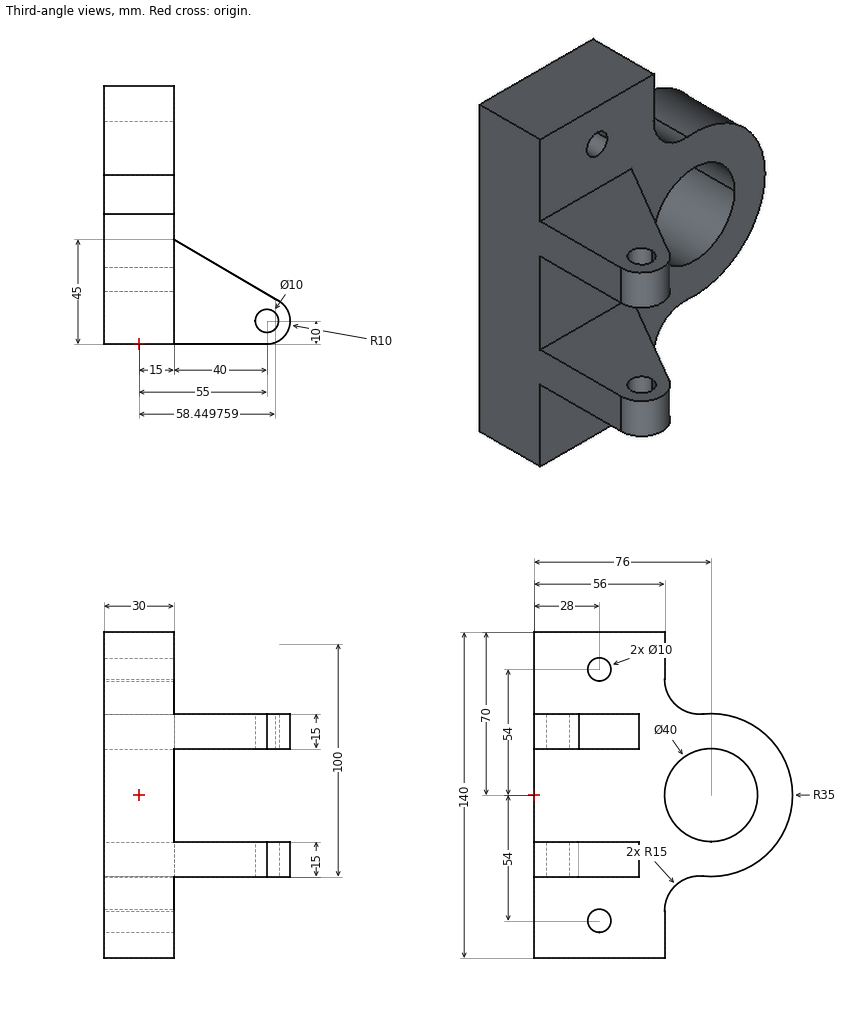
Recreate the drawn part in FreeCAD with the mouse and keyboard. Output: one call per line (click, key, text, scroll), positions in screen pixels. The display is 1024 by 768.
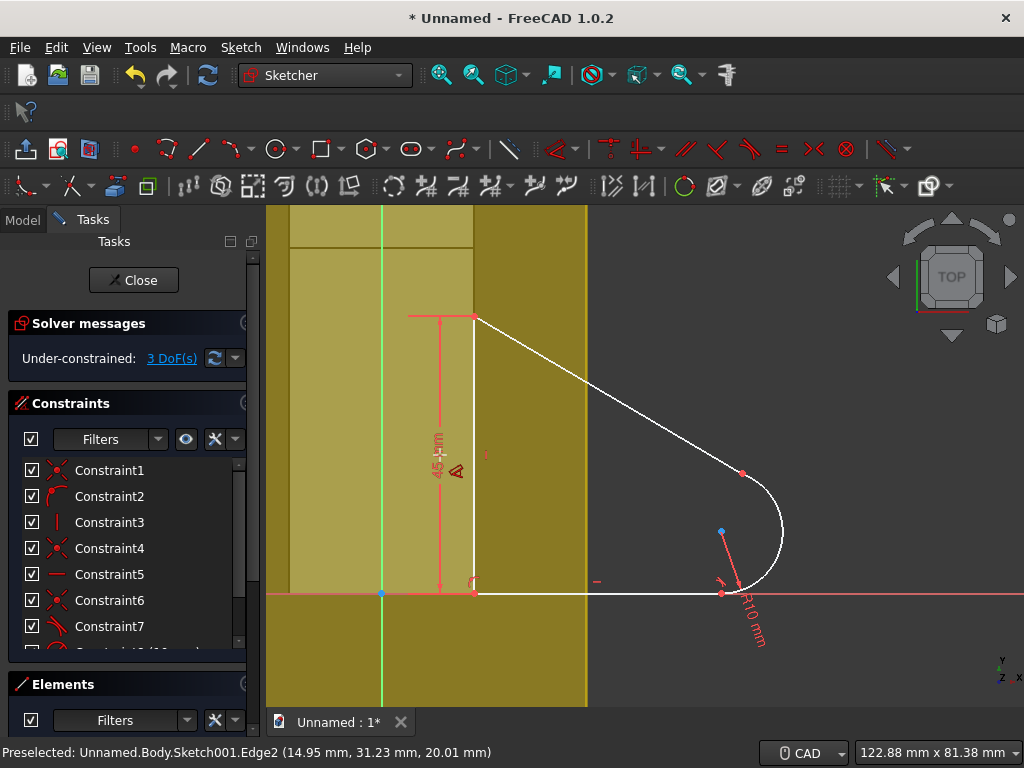
click(548, 594)
click(598, 628)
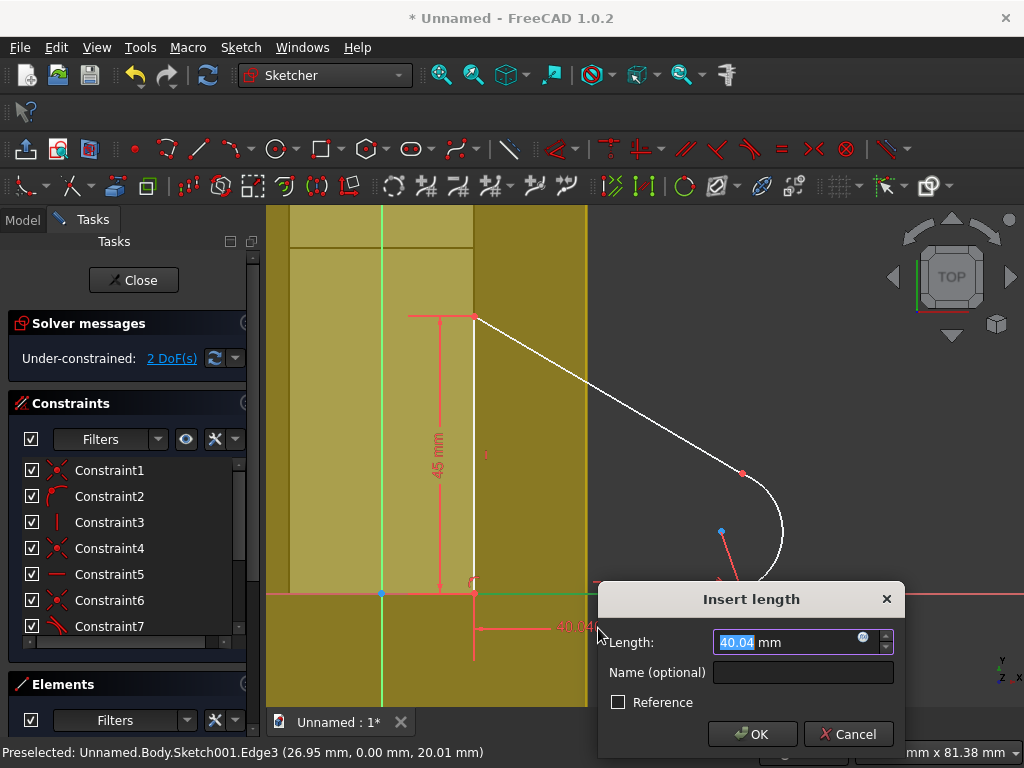
text(40)
key(Return)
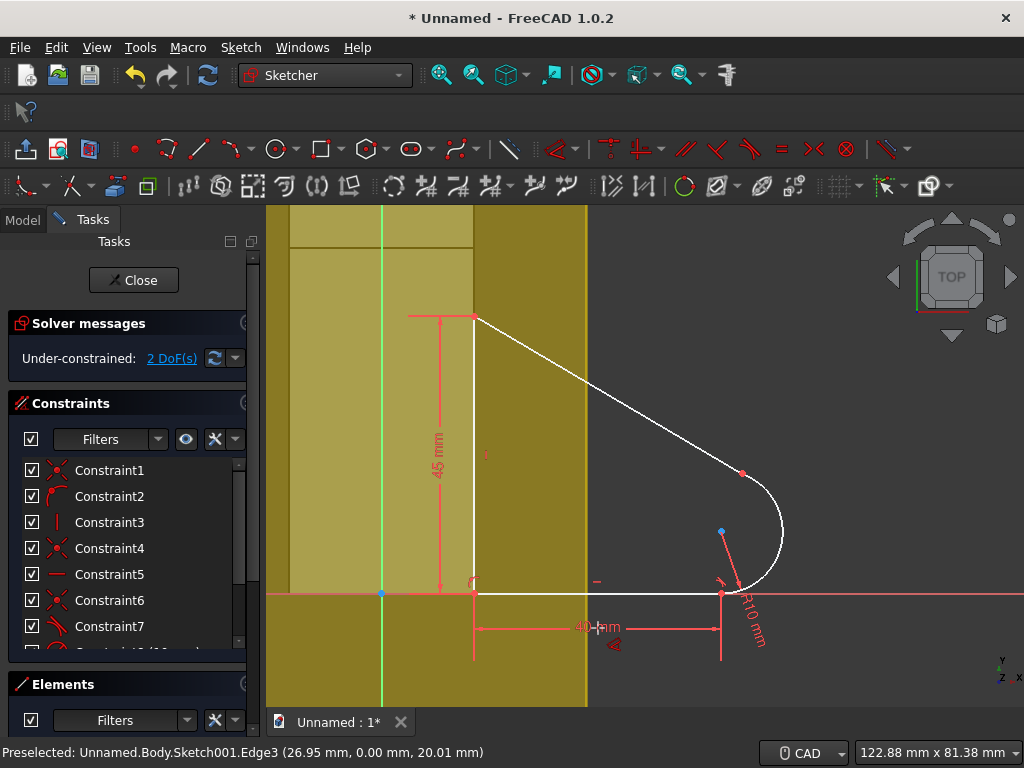
click(474, 316)
click(428, 628)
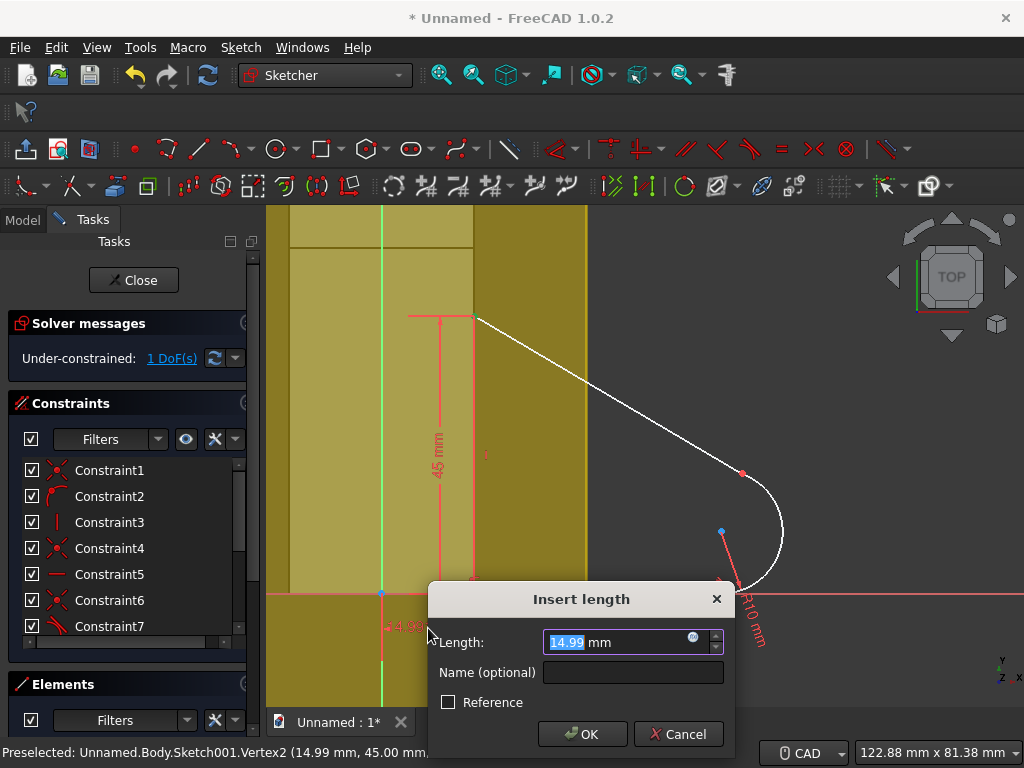
text(15)
key(Return)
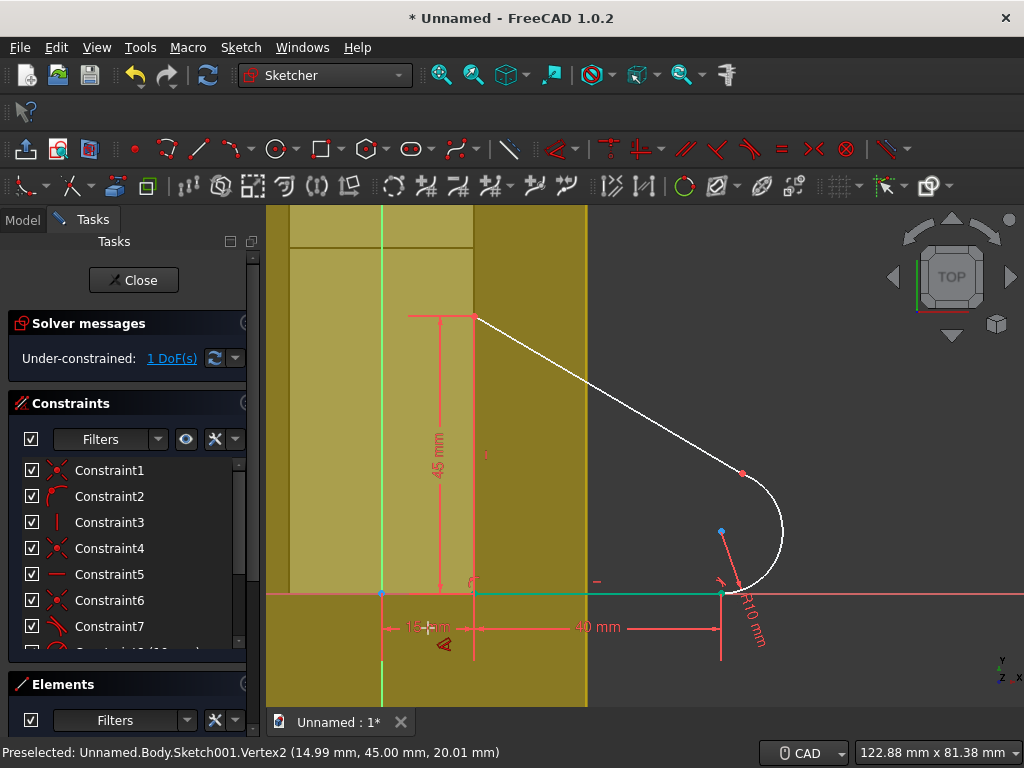
click(742, 474)
click(562, 440)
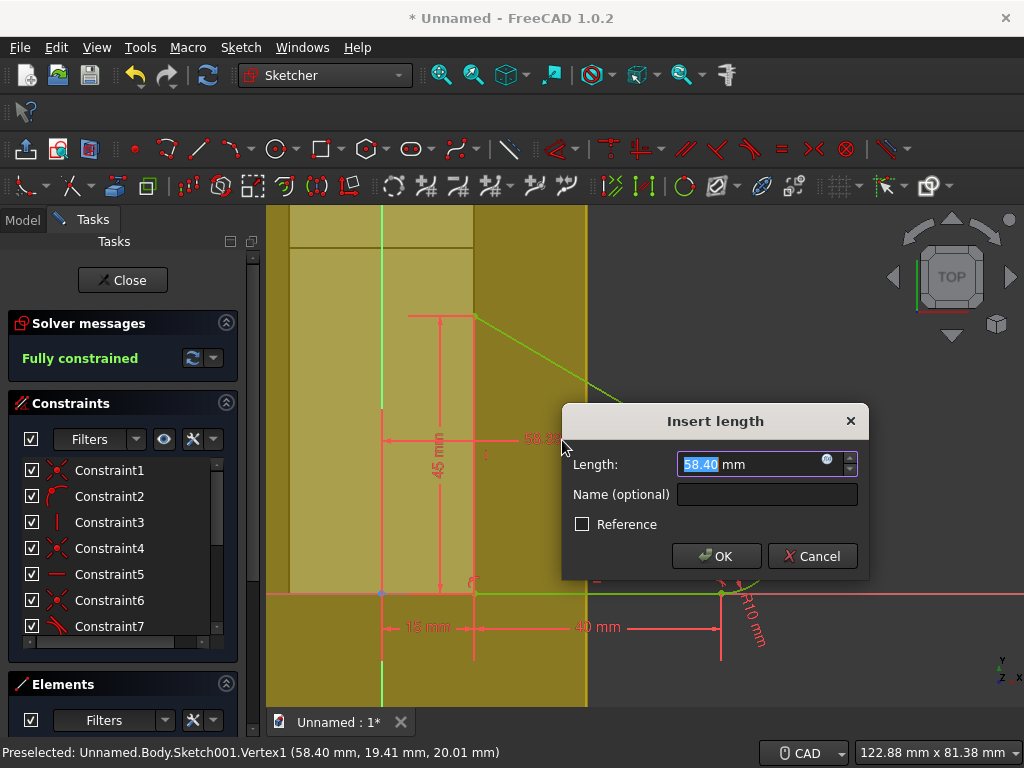
text(58.449759)
key(Return)
key(Escape)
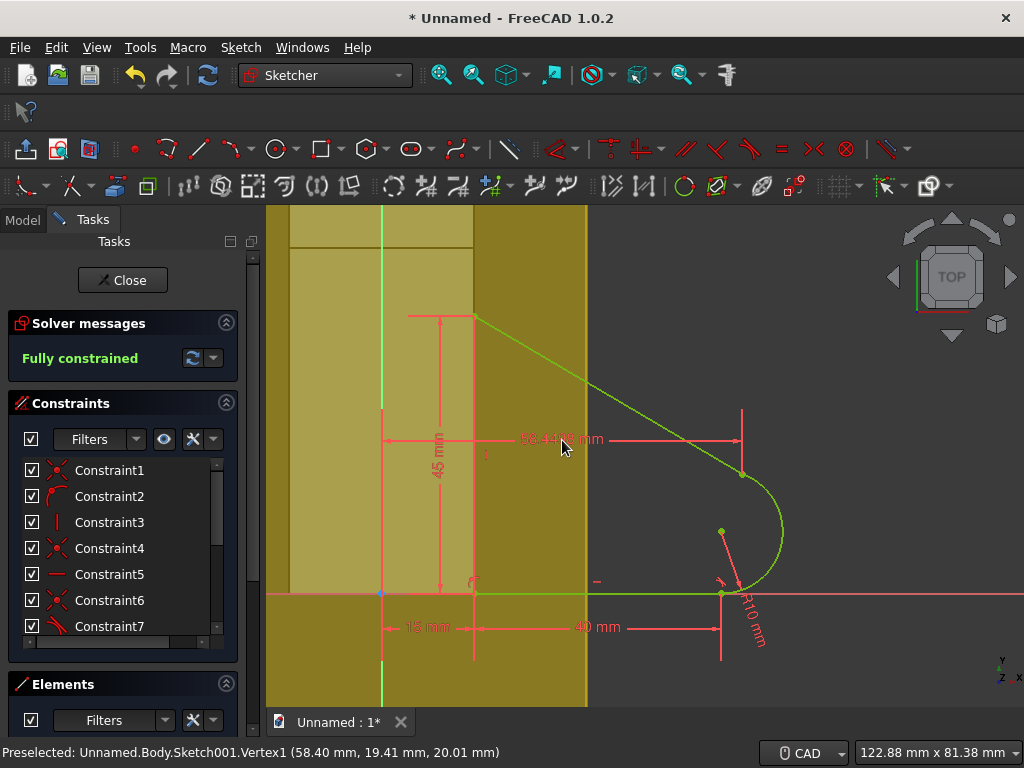
click(123, 280)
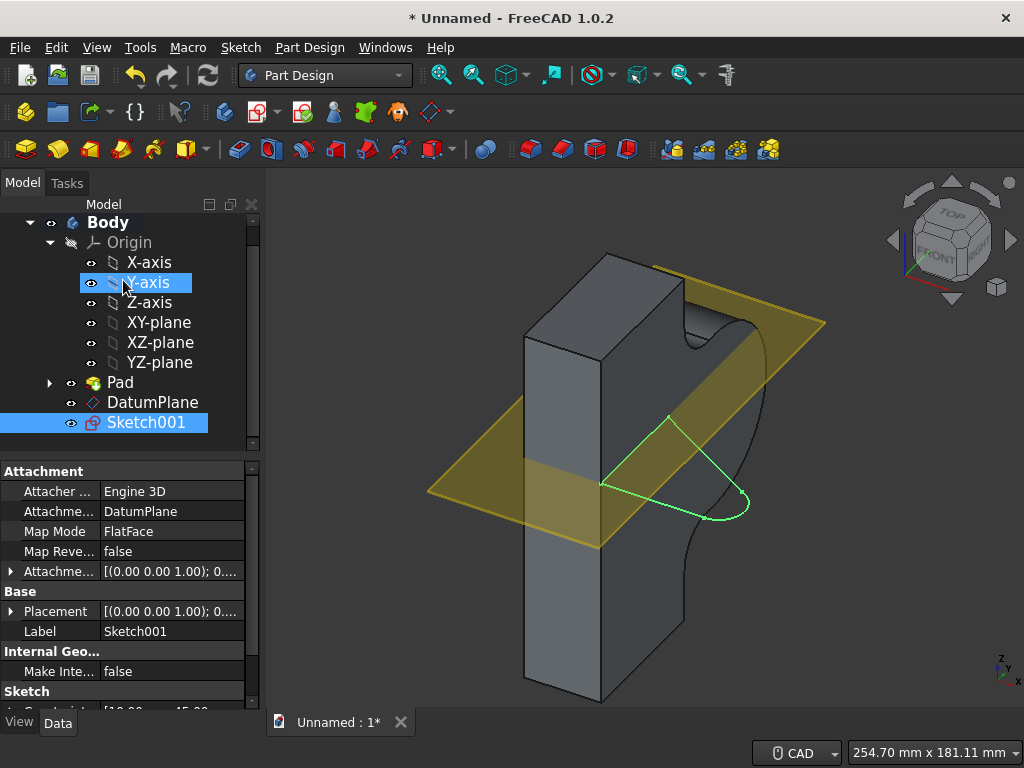
click(26, 150)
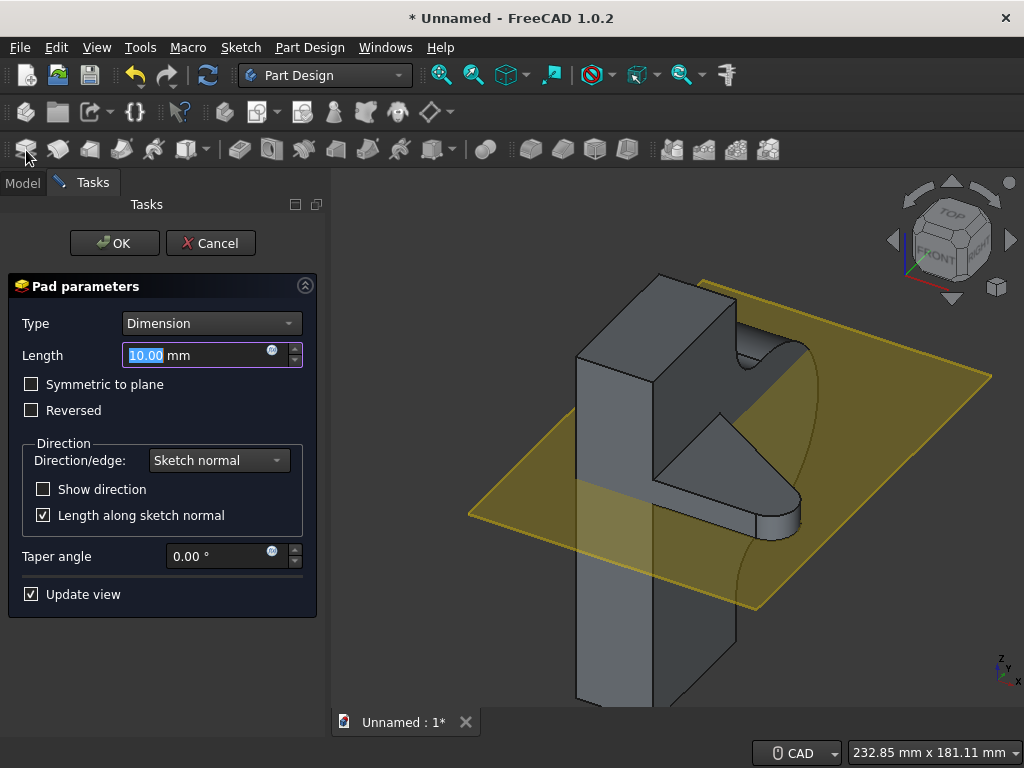
text(15)
key(Tab)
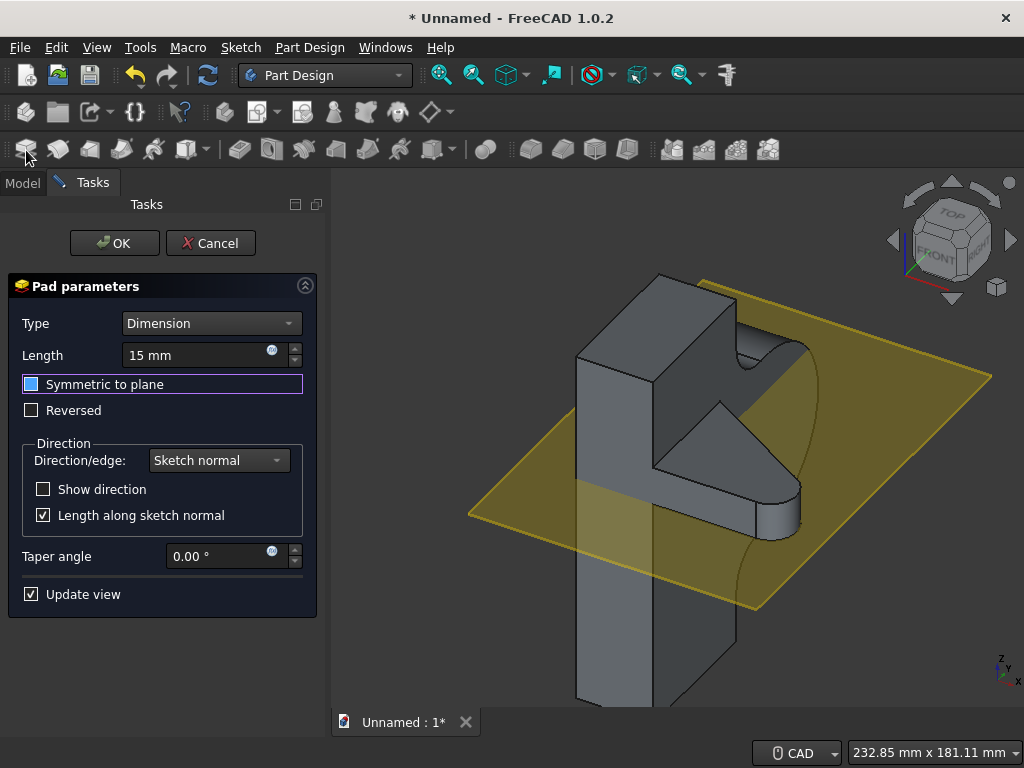
click(115, 243)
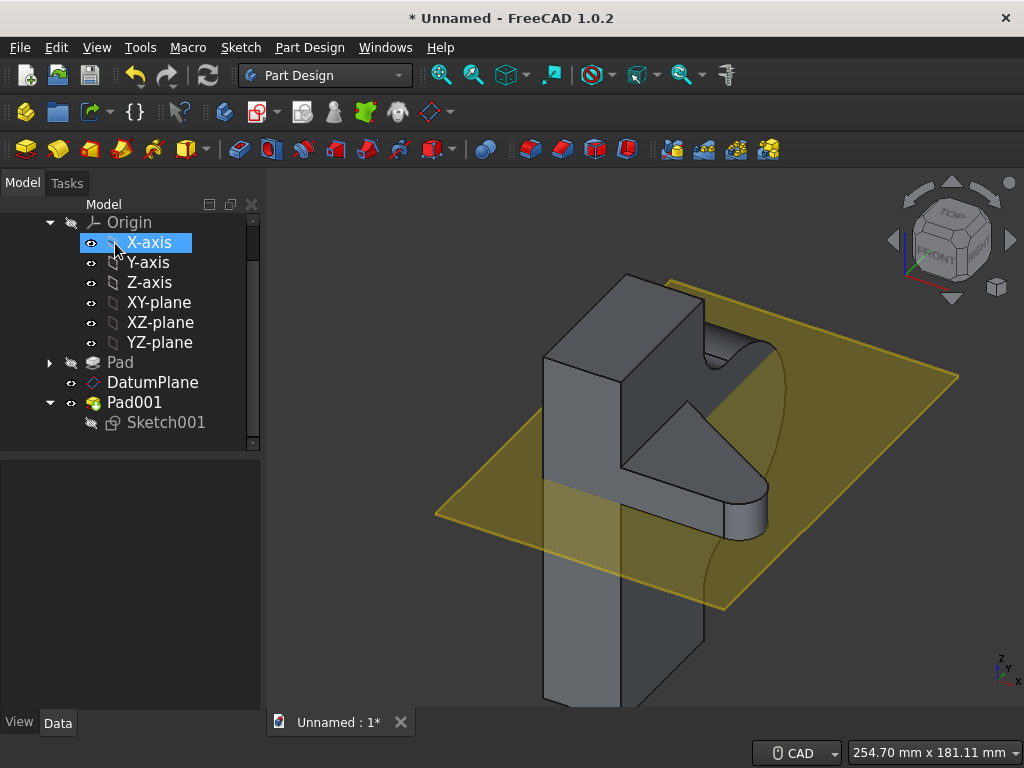
click(116, 383)
key(space)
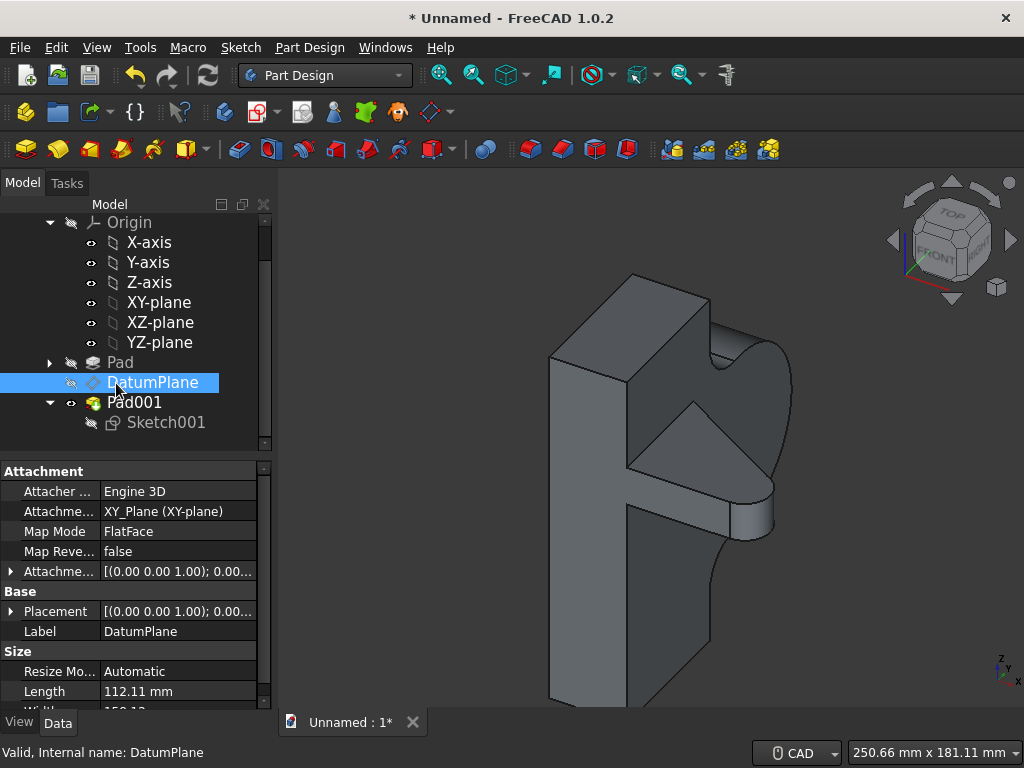
key(v)
key(f)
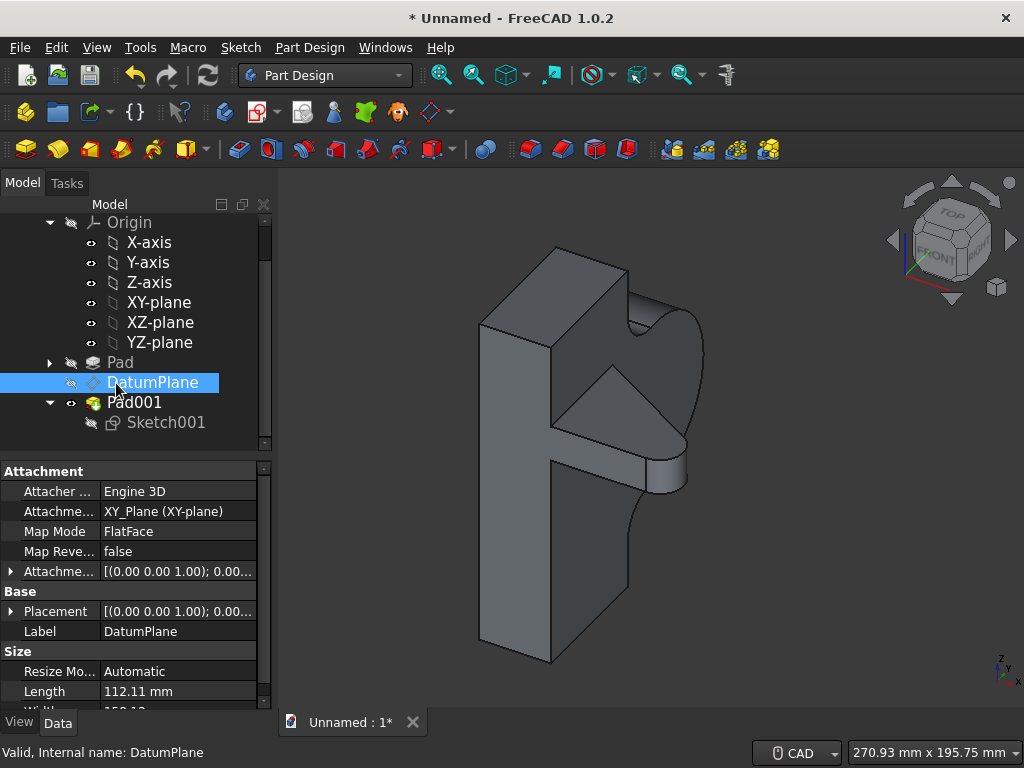
click(136, 303)